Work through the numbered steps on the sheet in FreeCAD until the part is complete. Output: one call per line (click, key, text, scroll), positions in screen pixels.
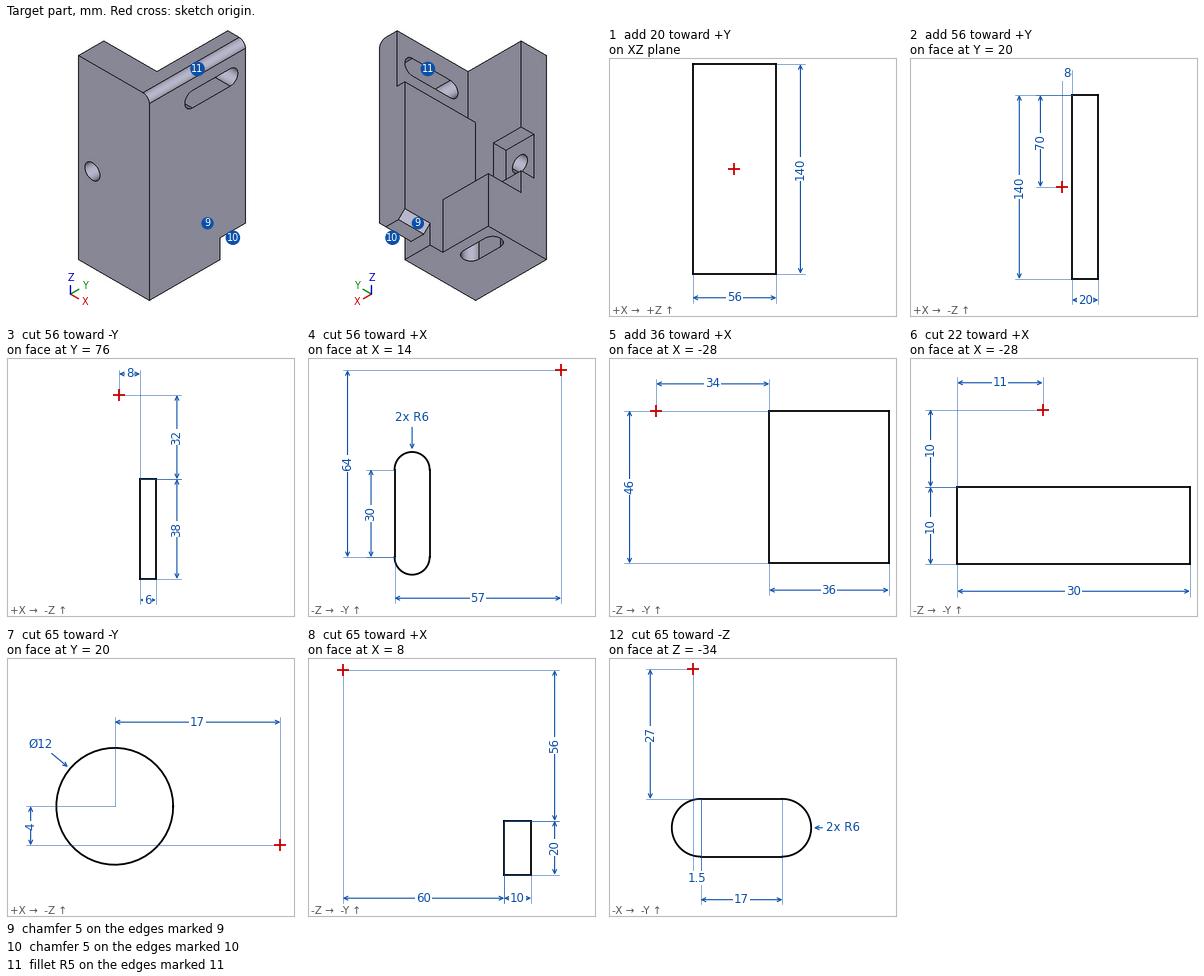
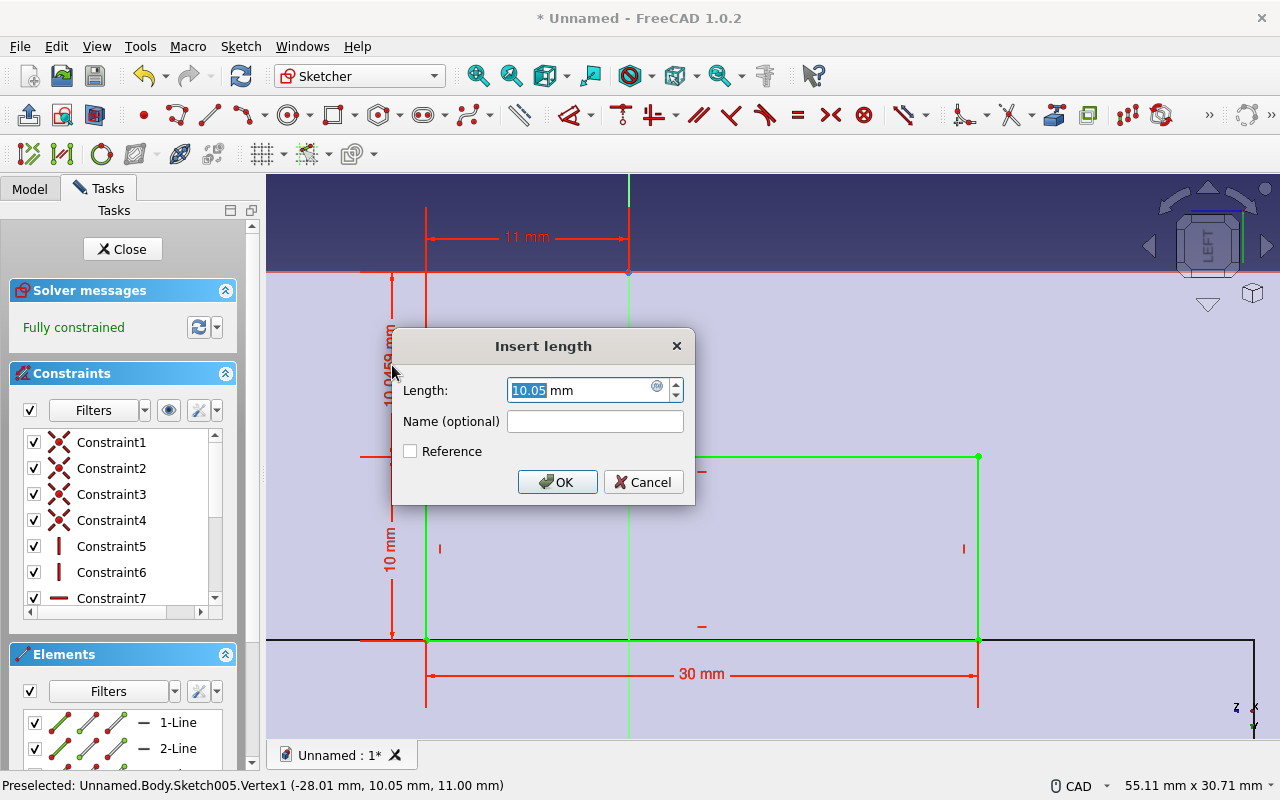
text(10)
key(Return)
key(Escape)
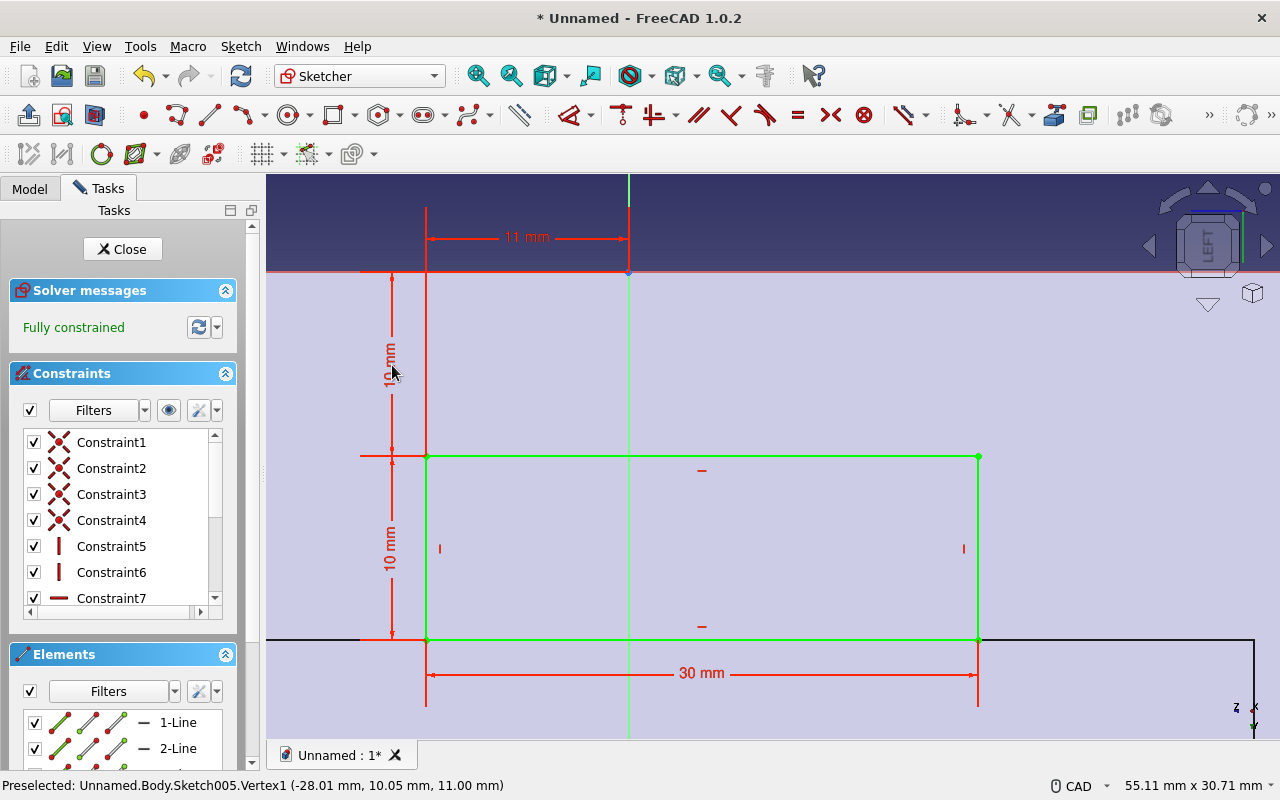
click(123, 249)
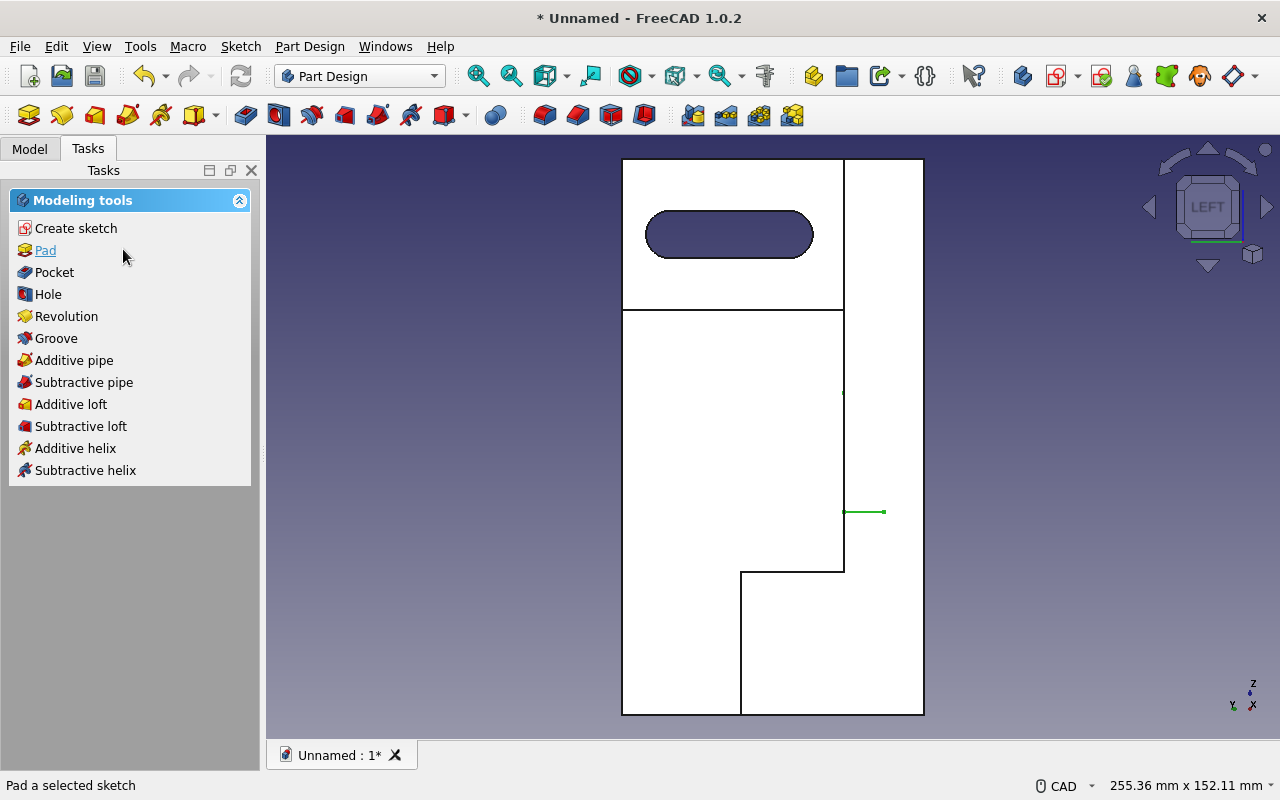
click(246, 116)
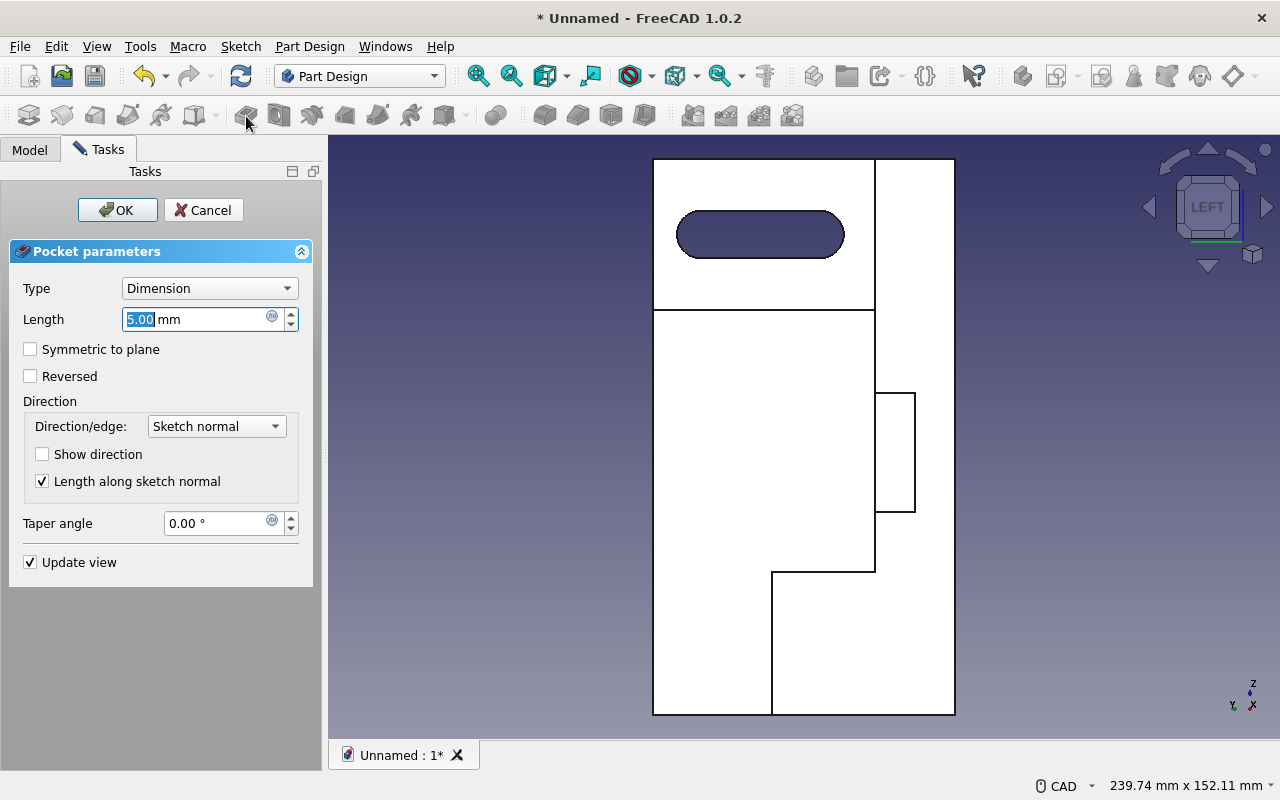
text(22)
key(Tab)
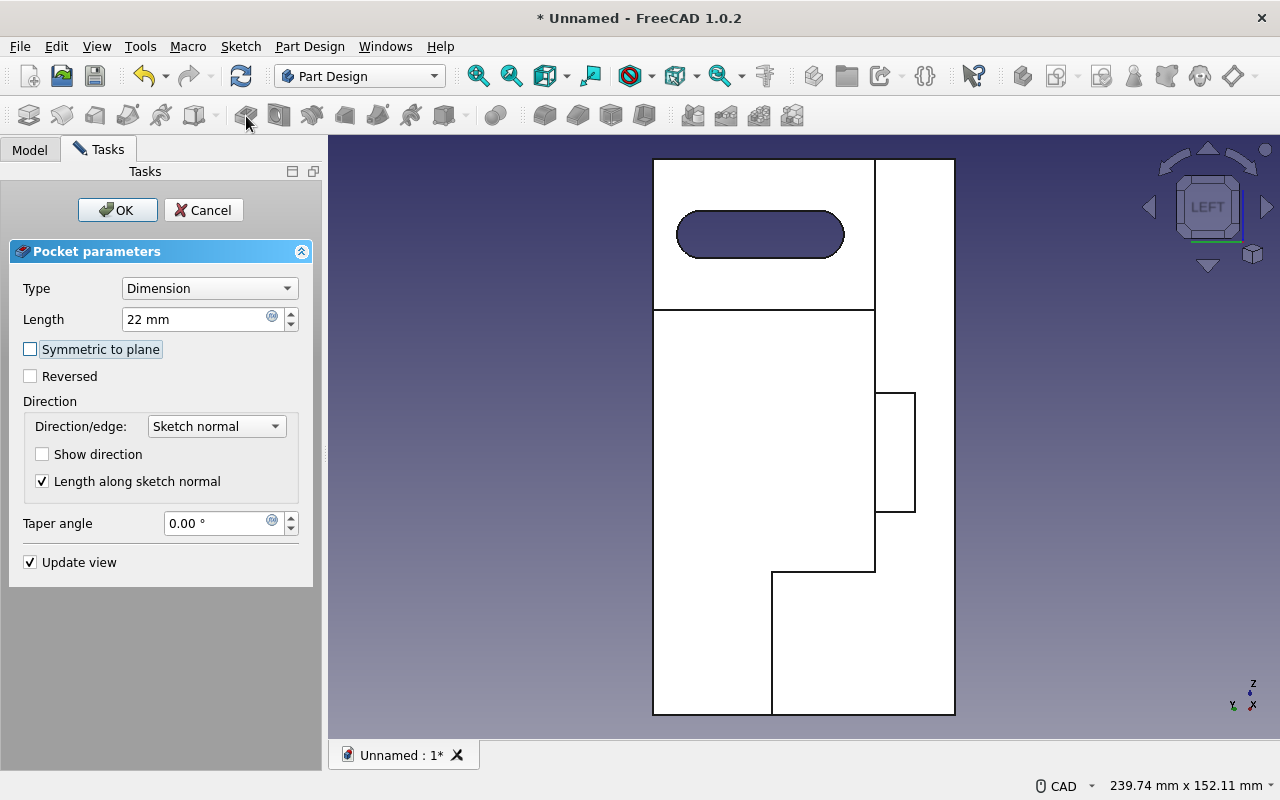
click(118, 210)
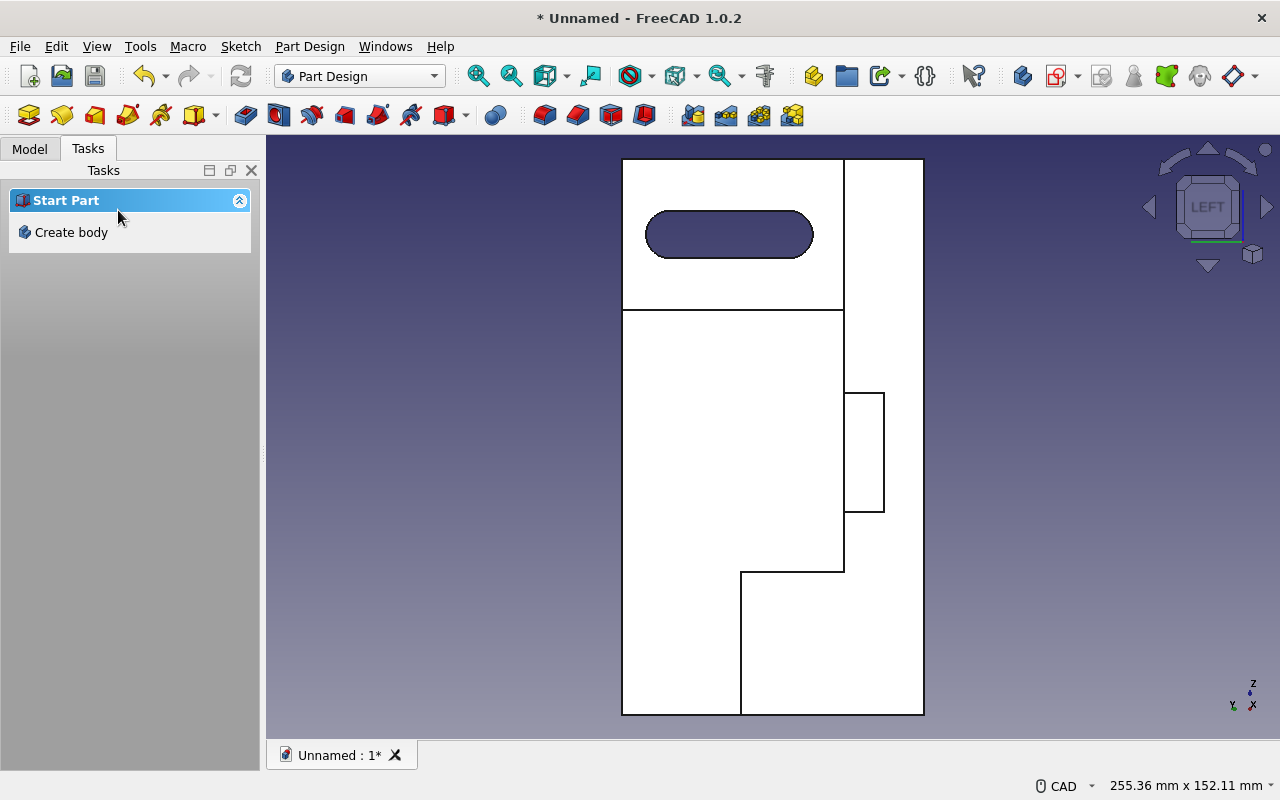
key(4)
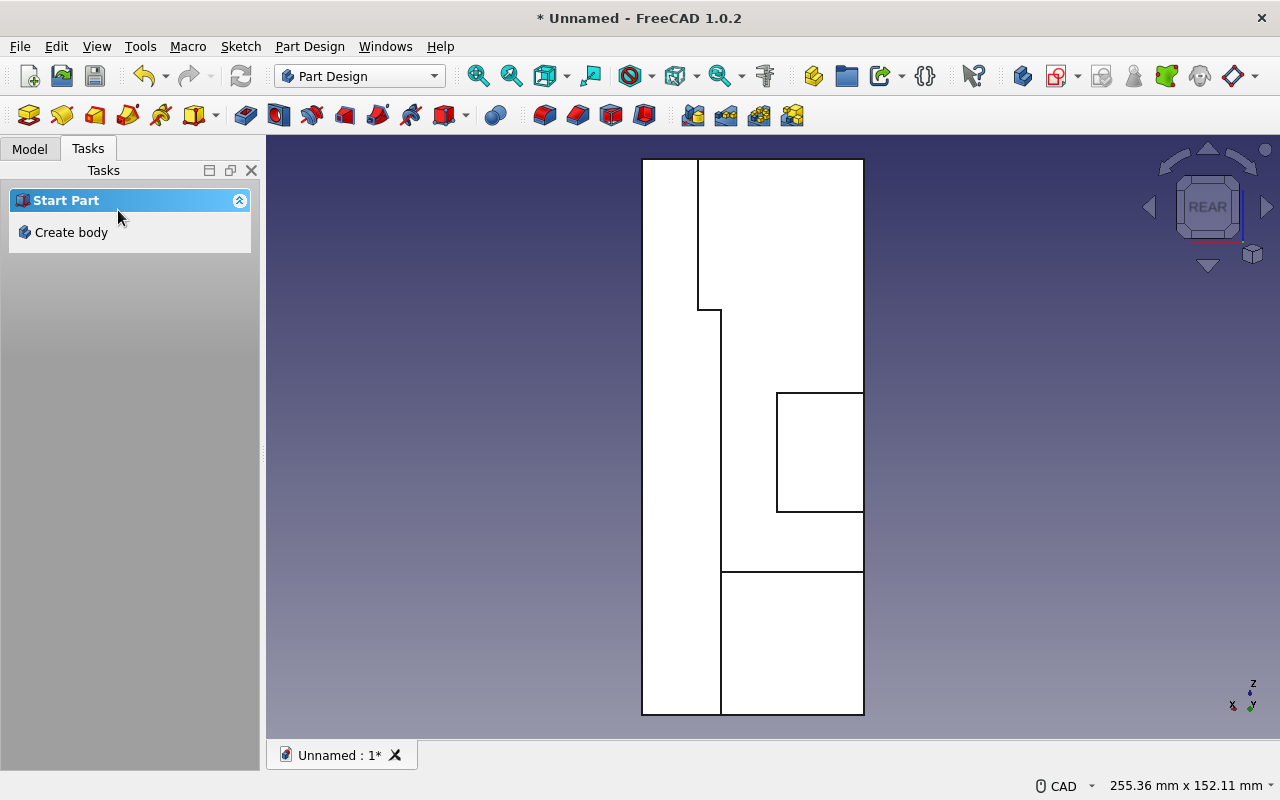
click(781, 247)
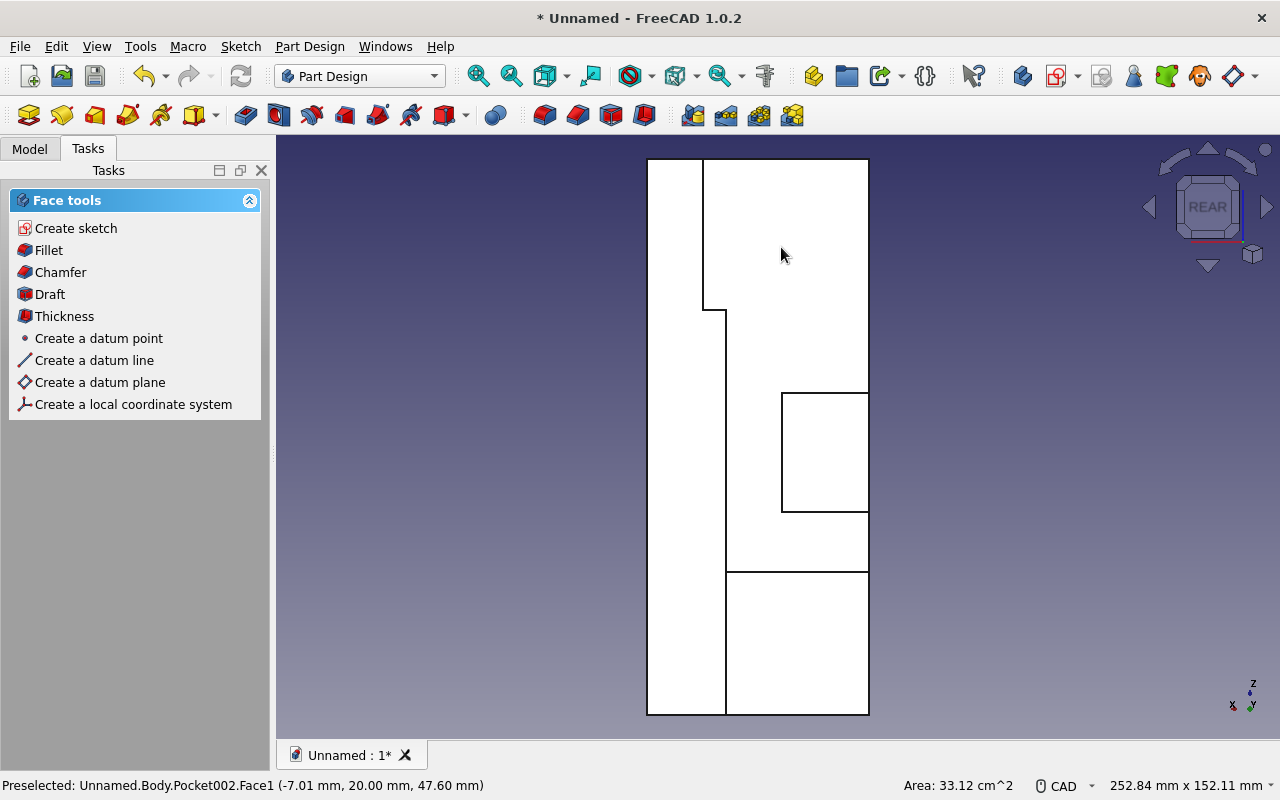
click(1056, 76)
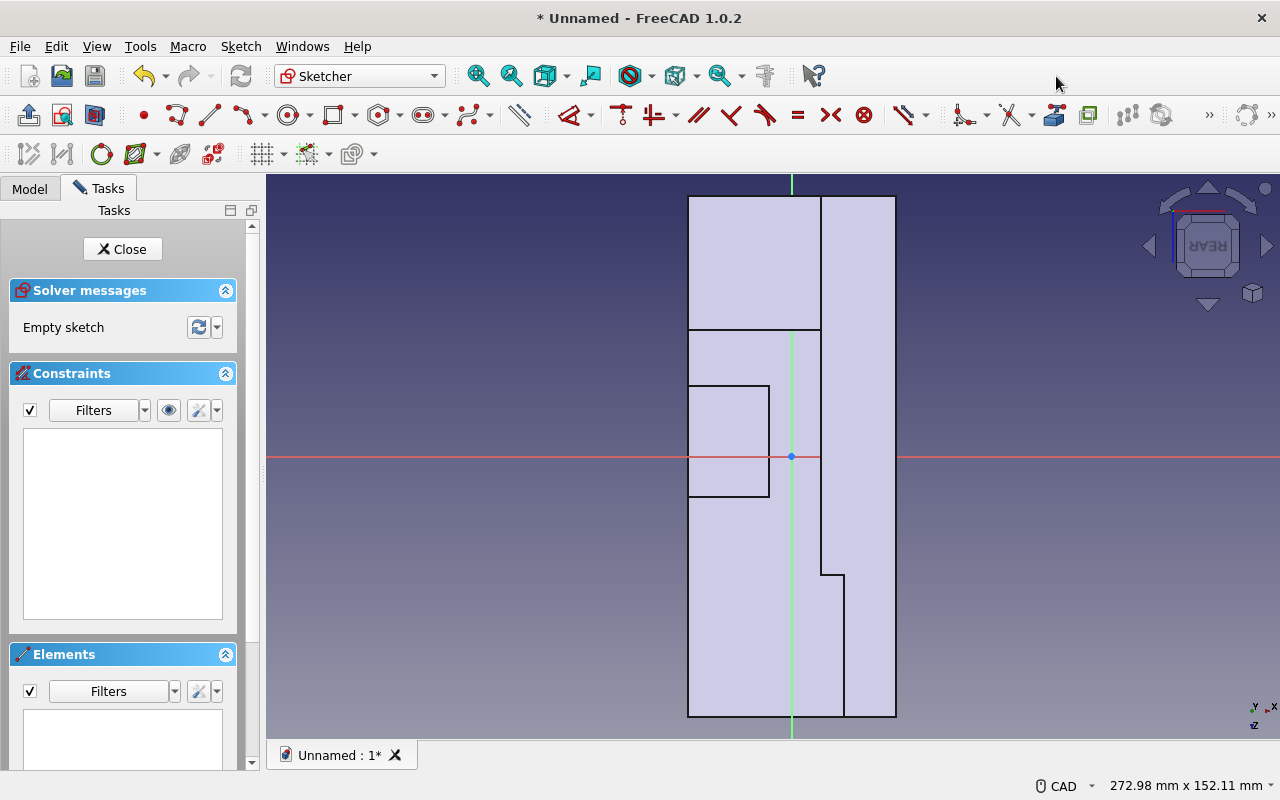
key(q)
key(s)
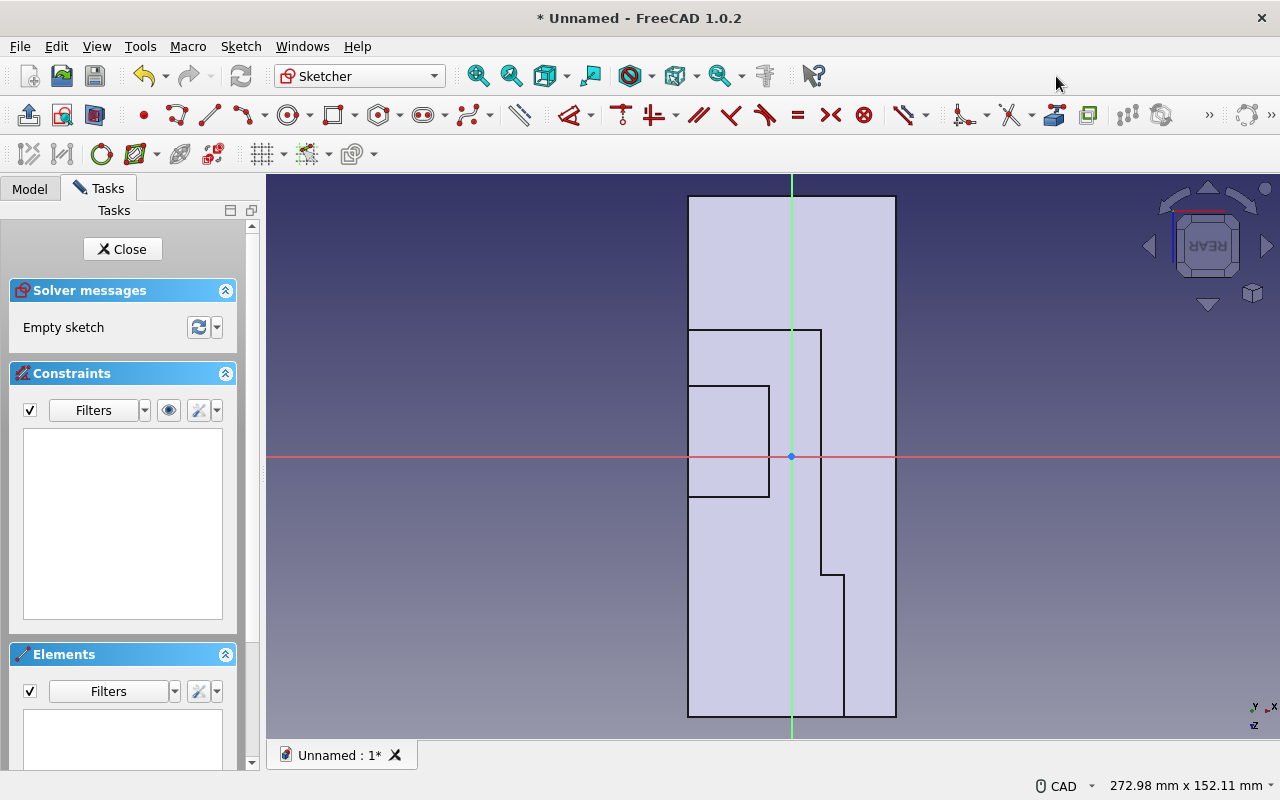
scroll(756, 439, up, 10)